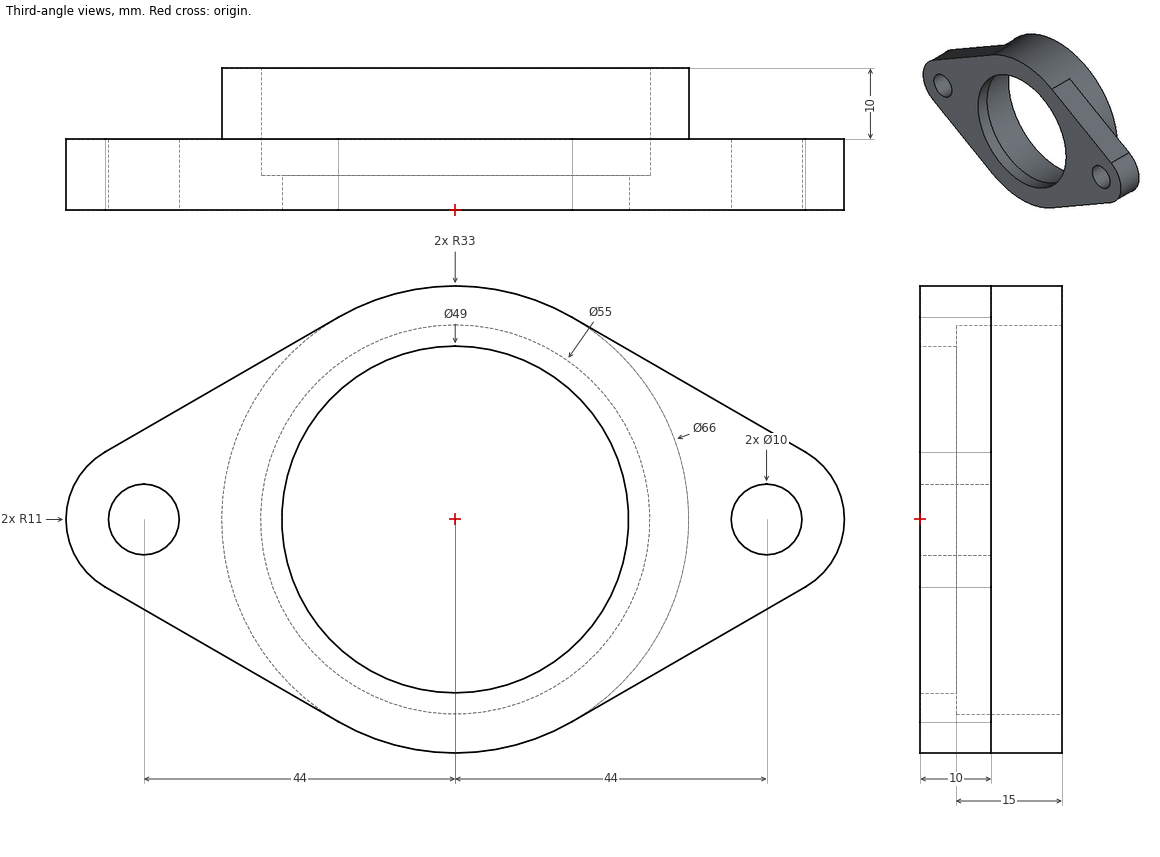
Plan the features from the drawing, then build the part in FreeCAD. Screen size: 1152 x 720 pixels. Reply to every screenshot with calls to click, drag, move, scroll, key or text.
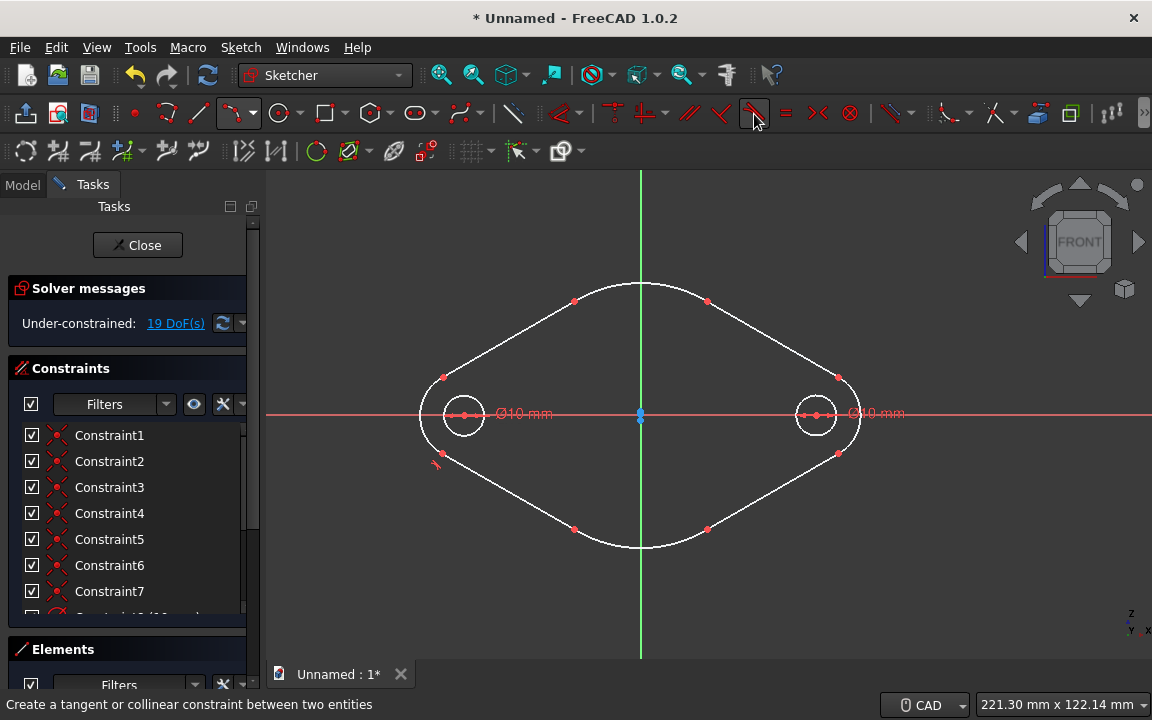
click(535, 507)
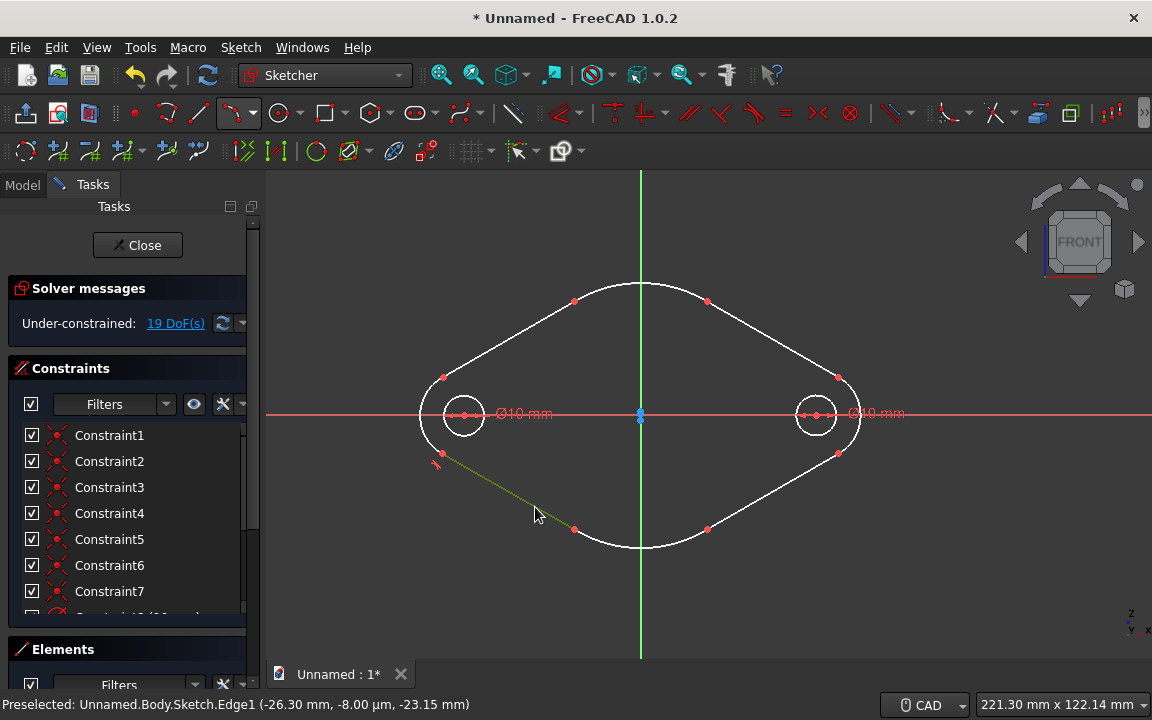
click(613, 545)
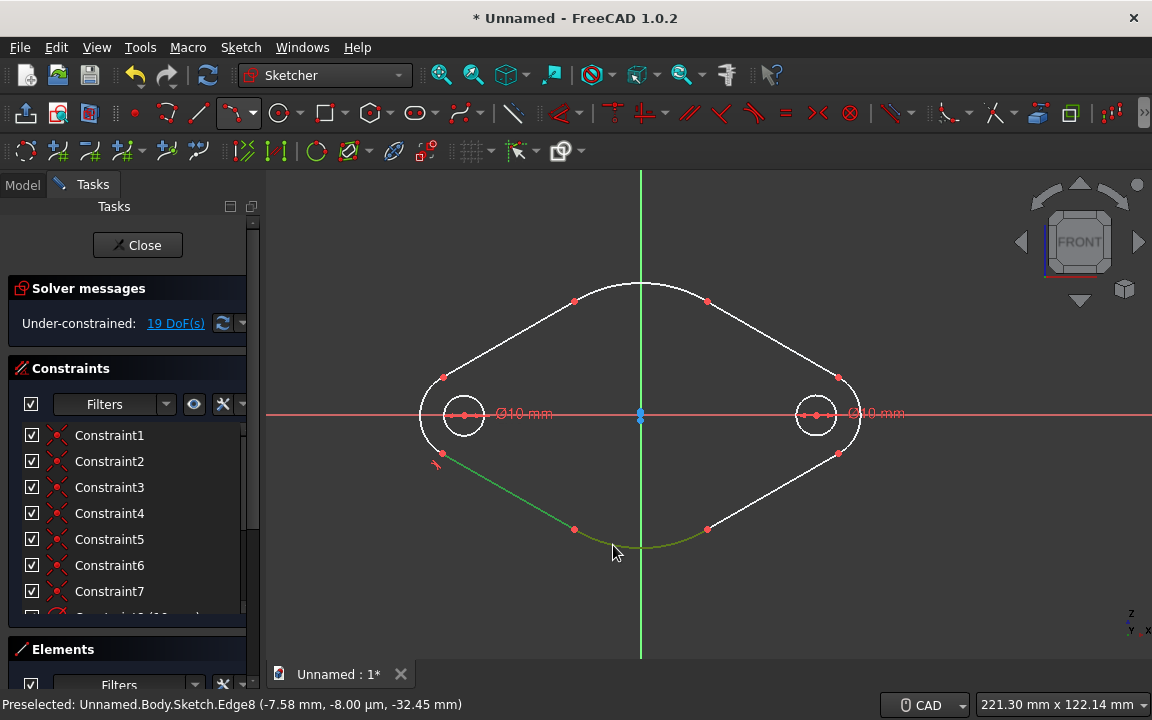
click(754, 114)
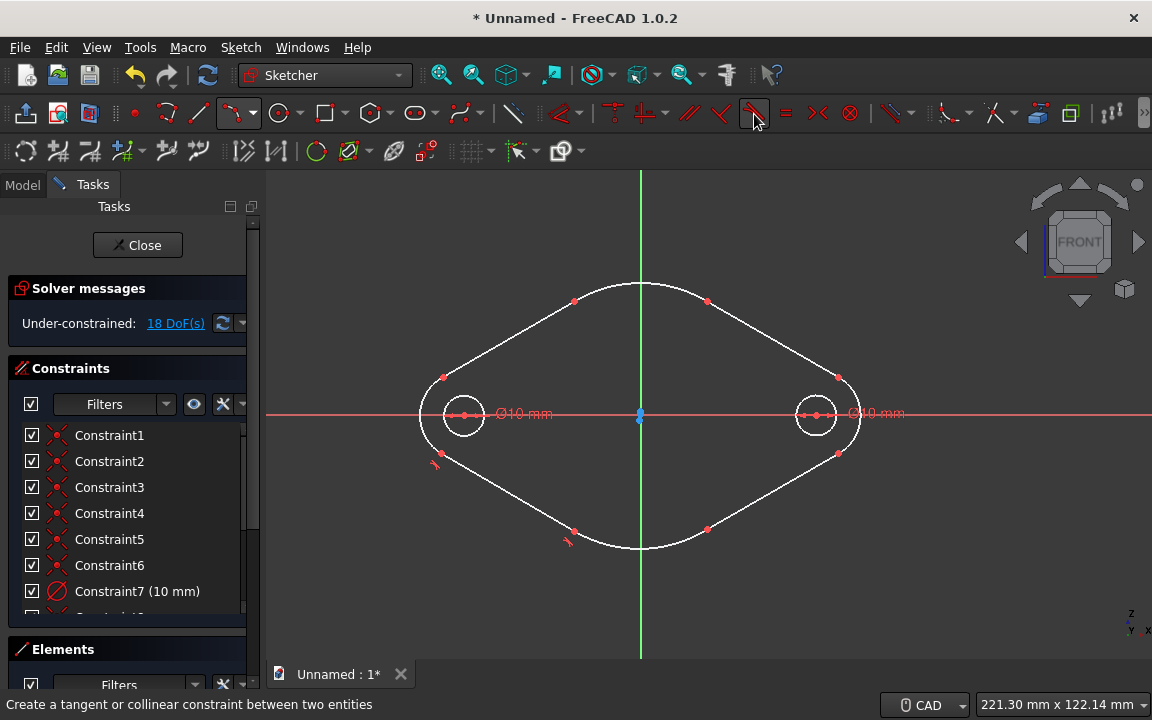
click(483, 354)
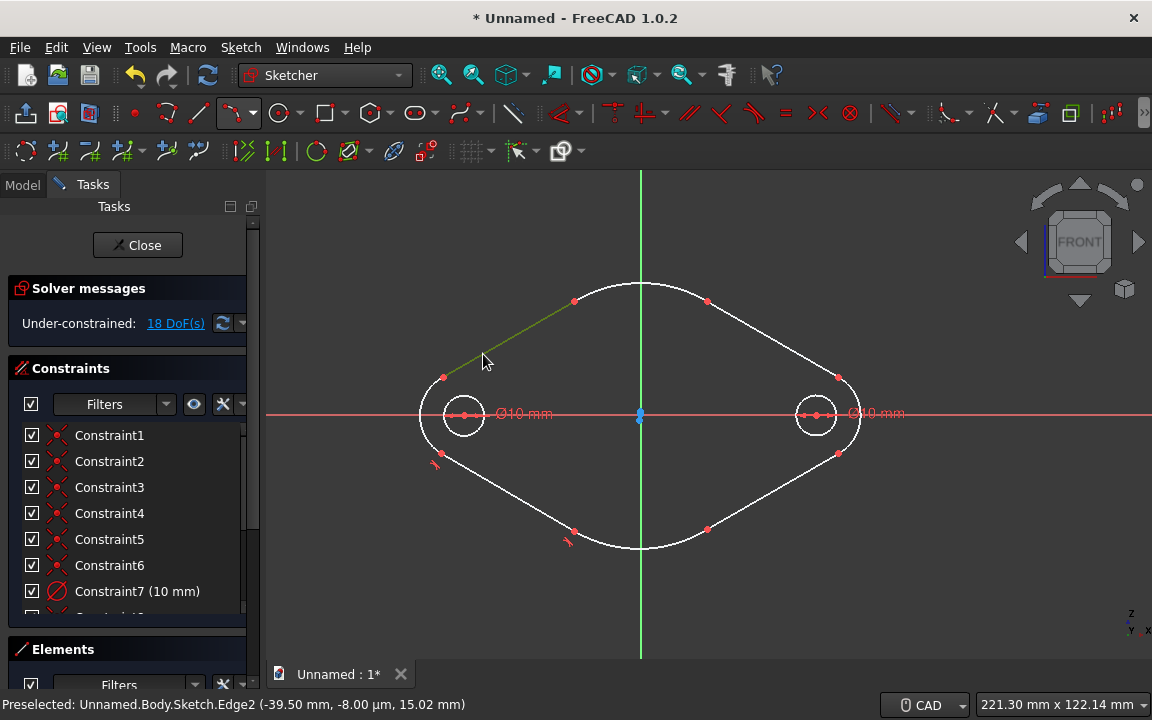
click(424, 397)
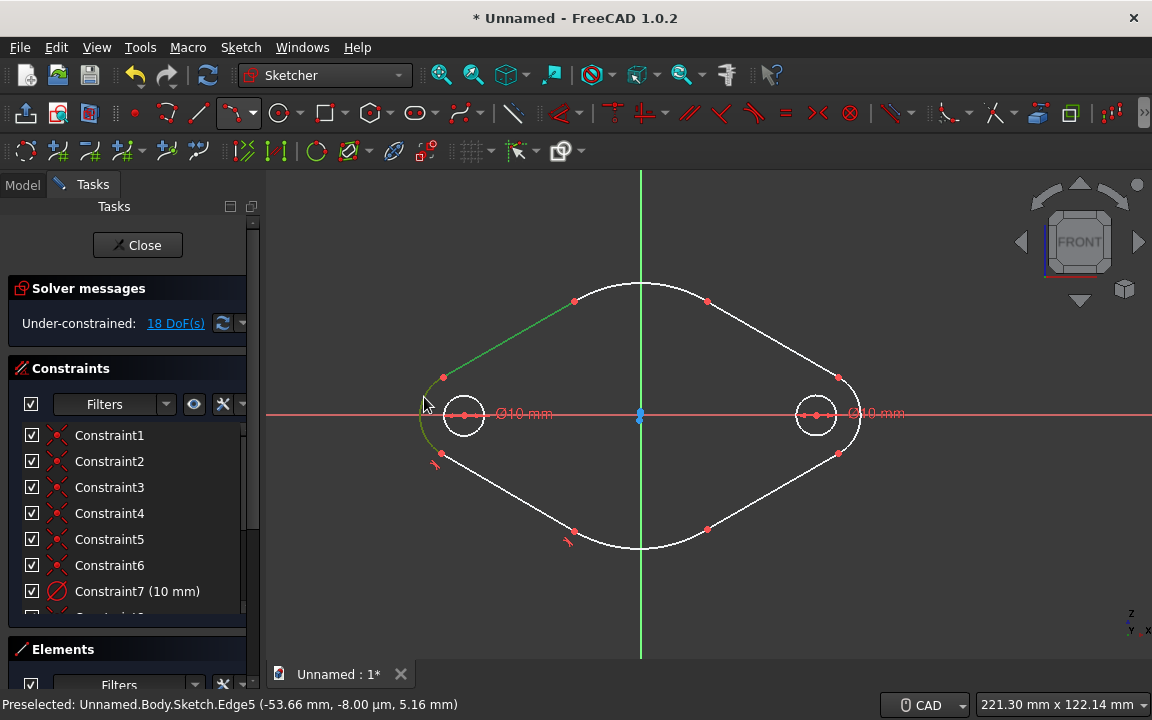
click(754, 114)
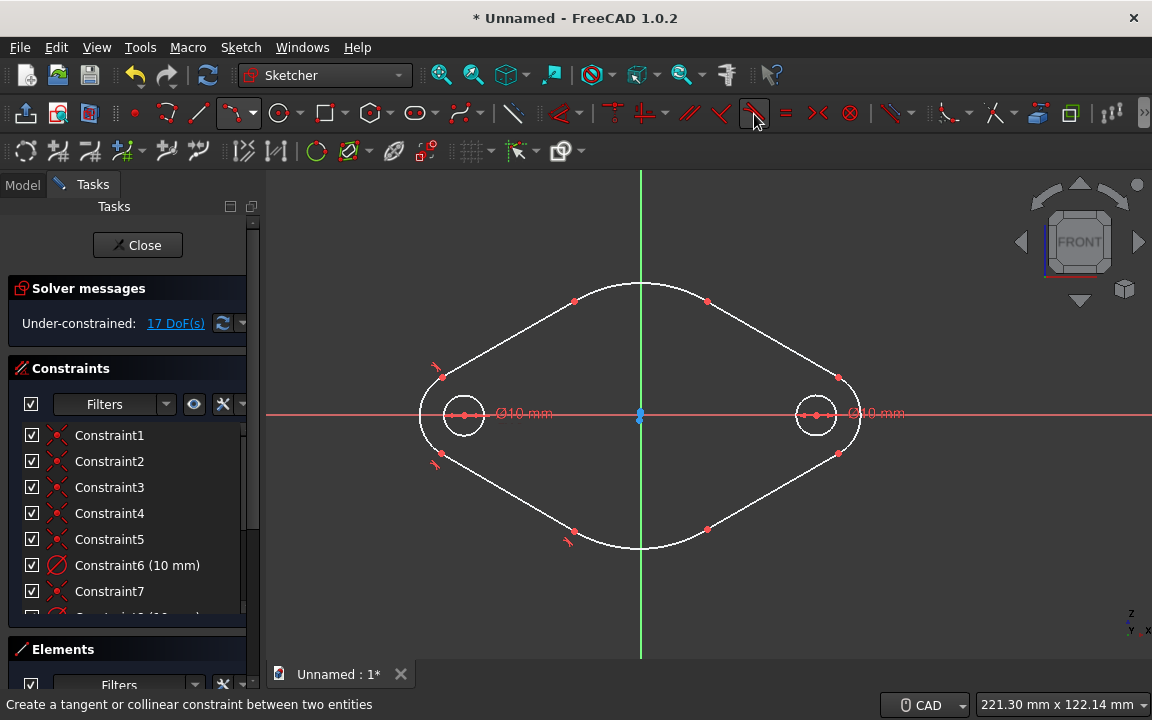
click(482, 354)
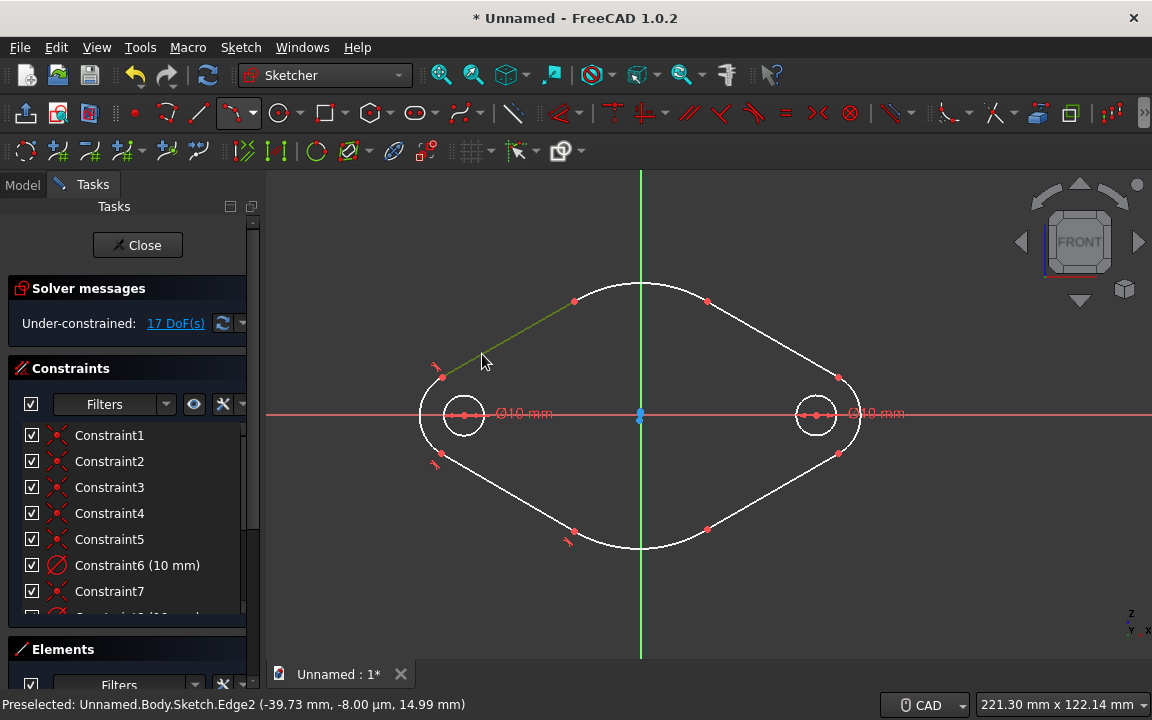
click(668, 286)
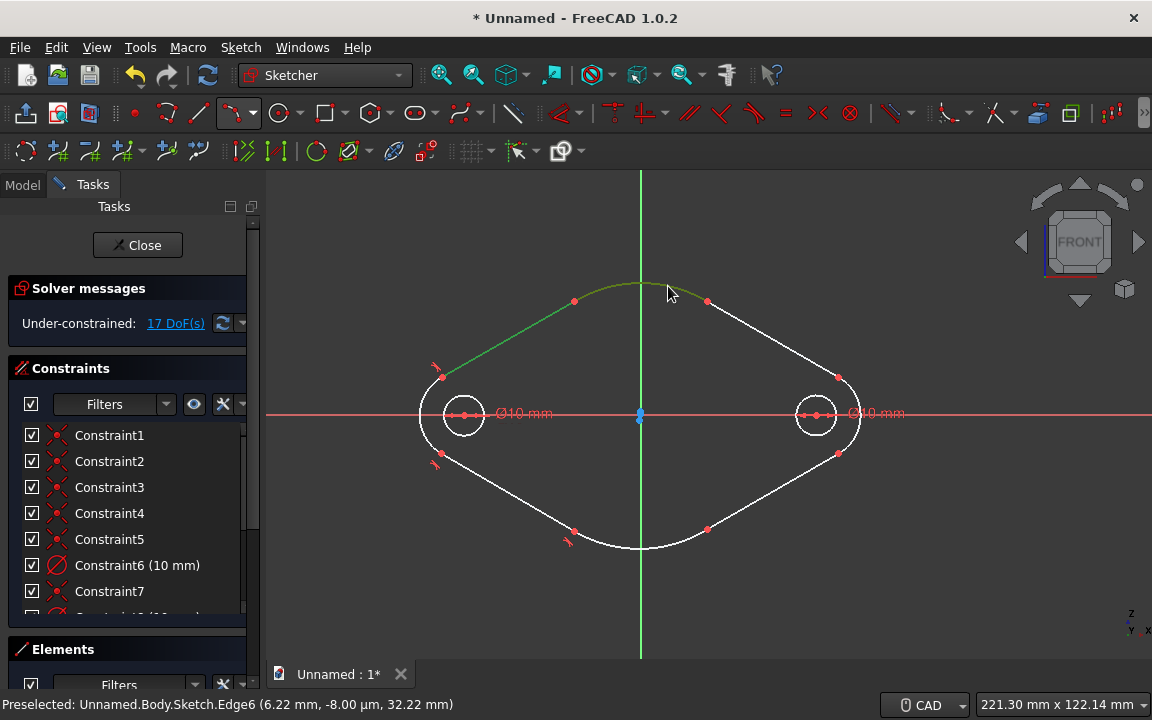
click(754, 114)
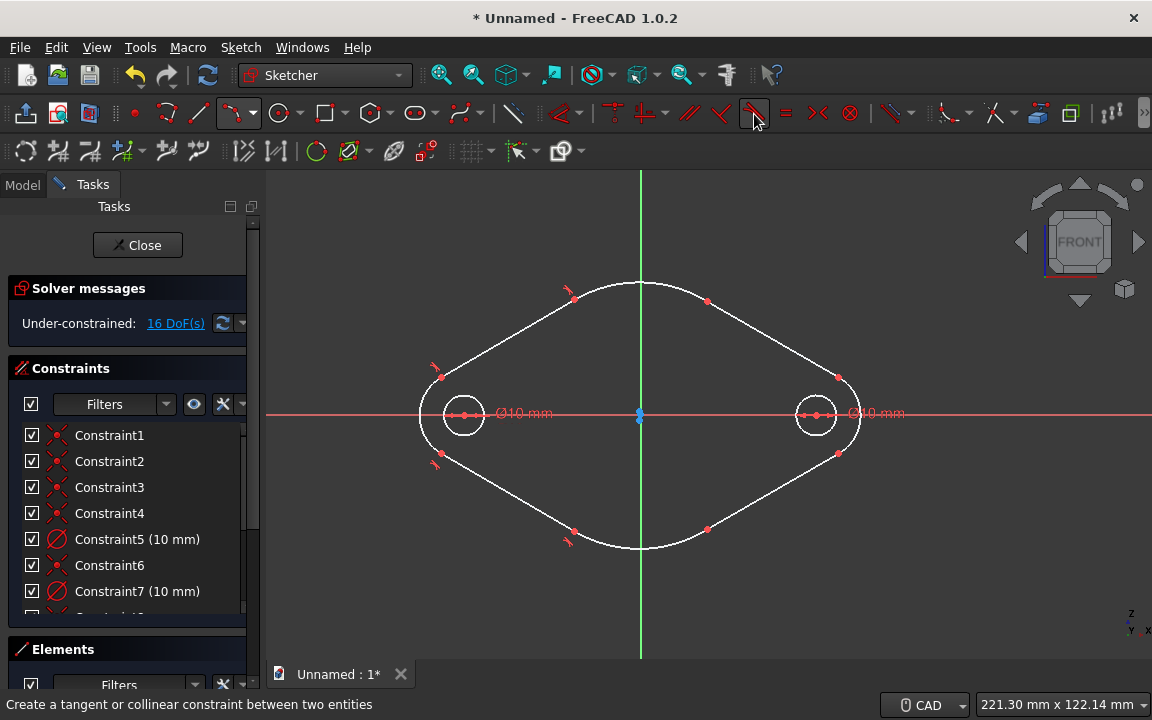
click(746, 324)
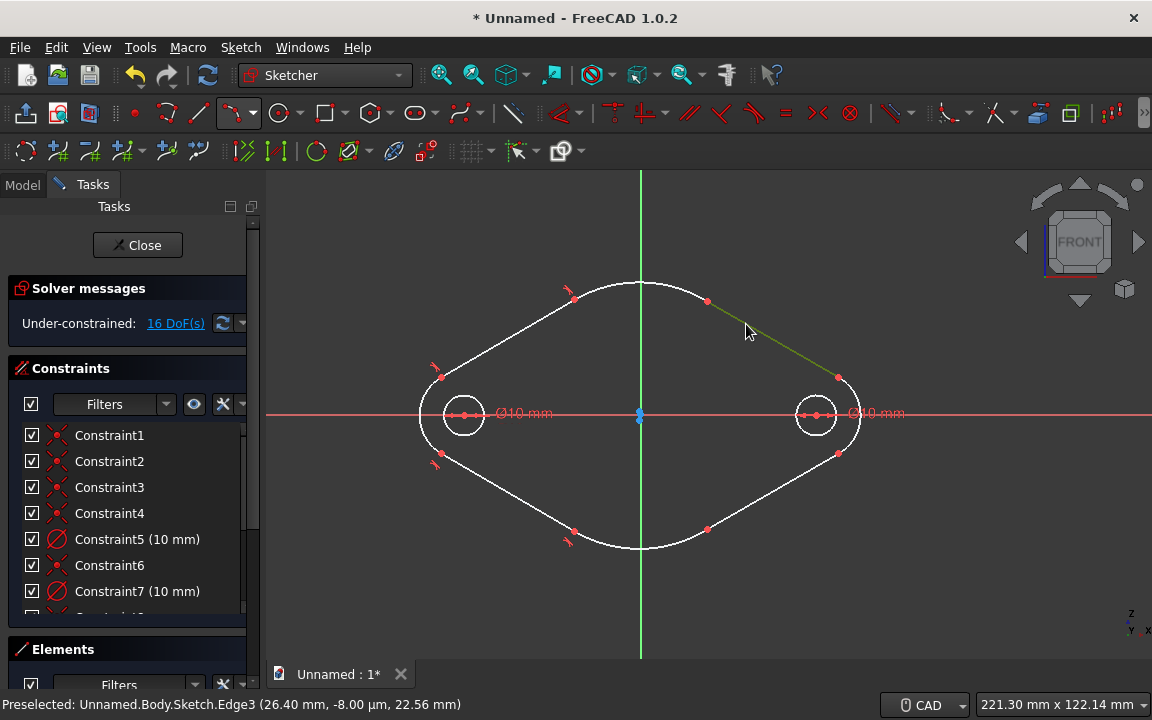
click(669, 286)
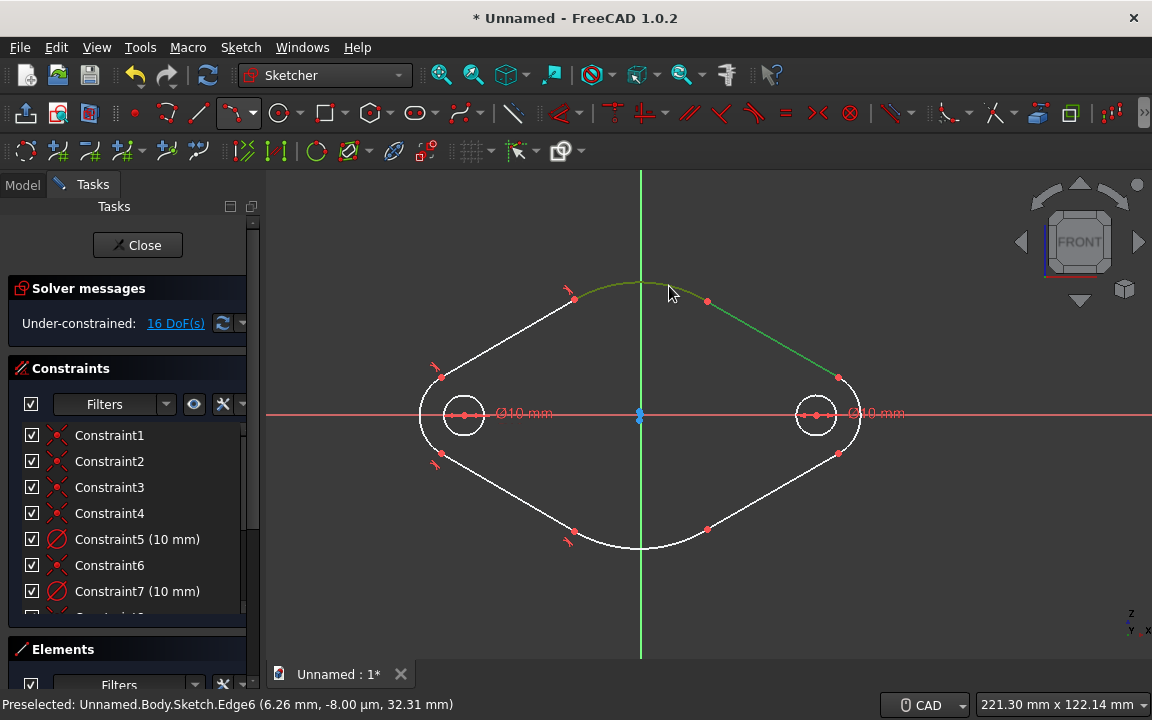
click(754, 114)